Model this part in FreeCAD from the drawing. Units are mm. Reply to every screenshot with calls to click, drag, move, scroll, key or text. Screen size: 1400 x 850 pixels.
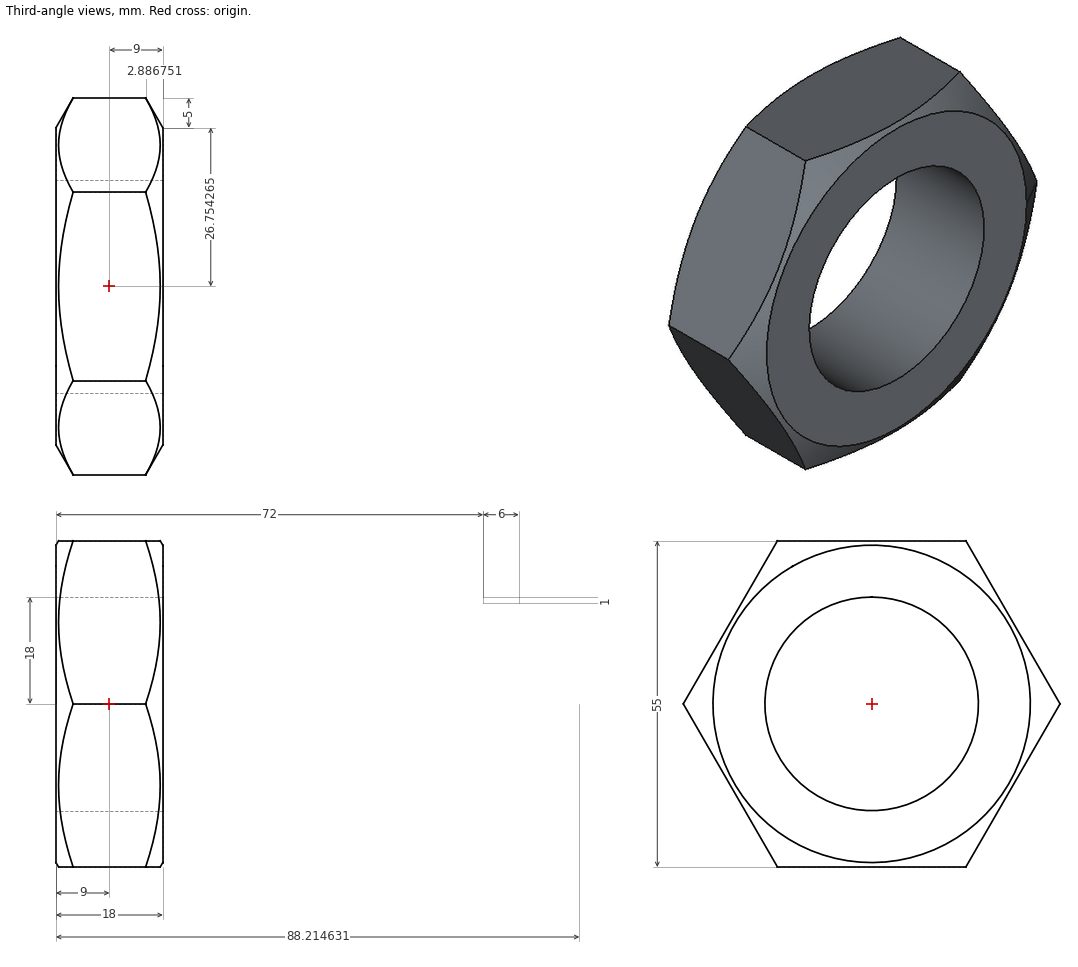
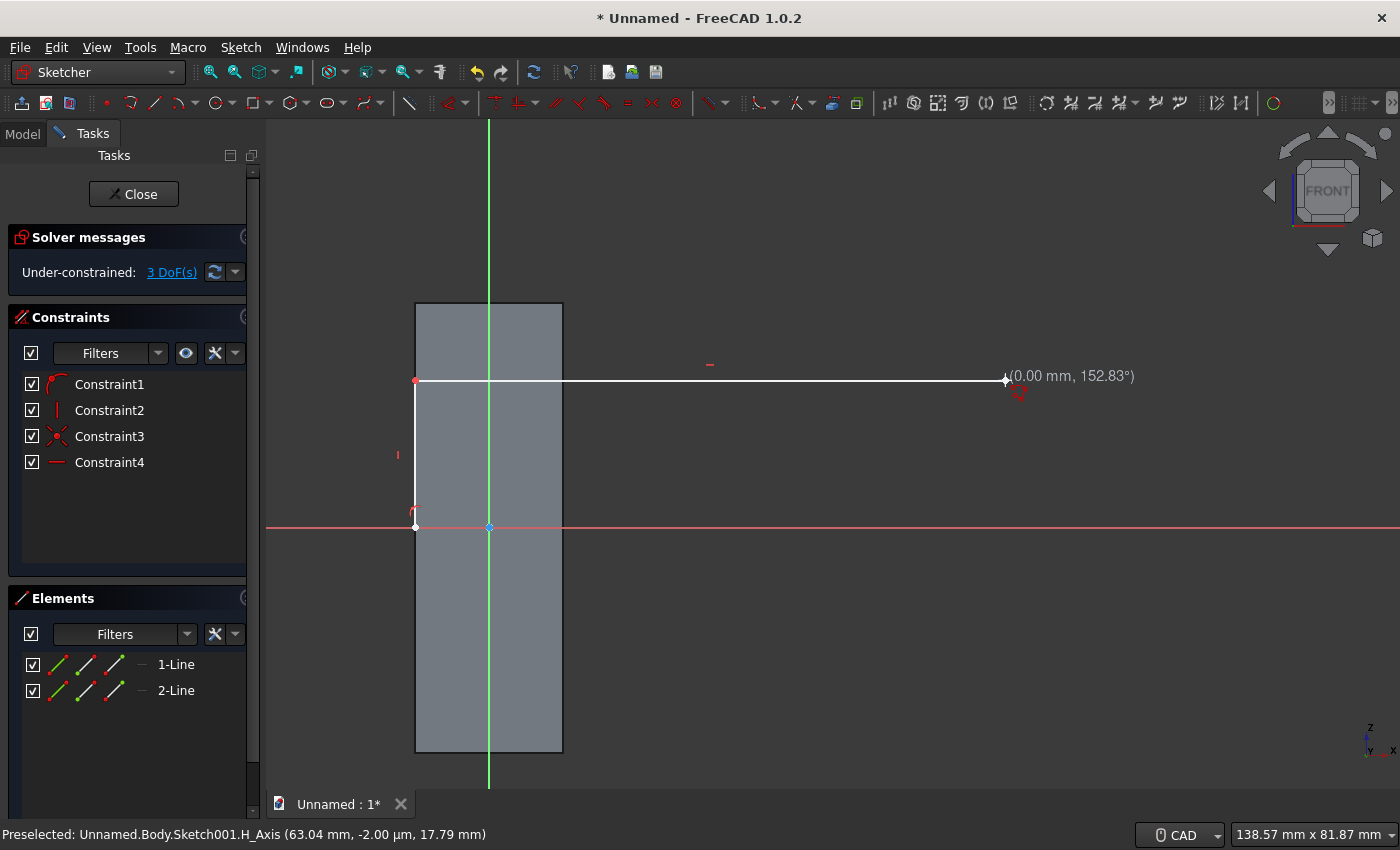
scroll(1005, 388, up, 4)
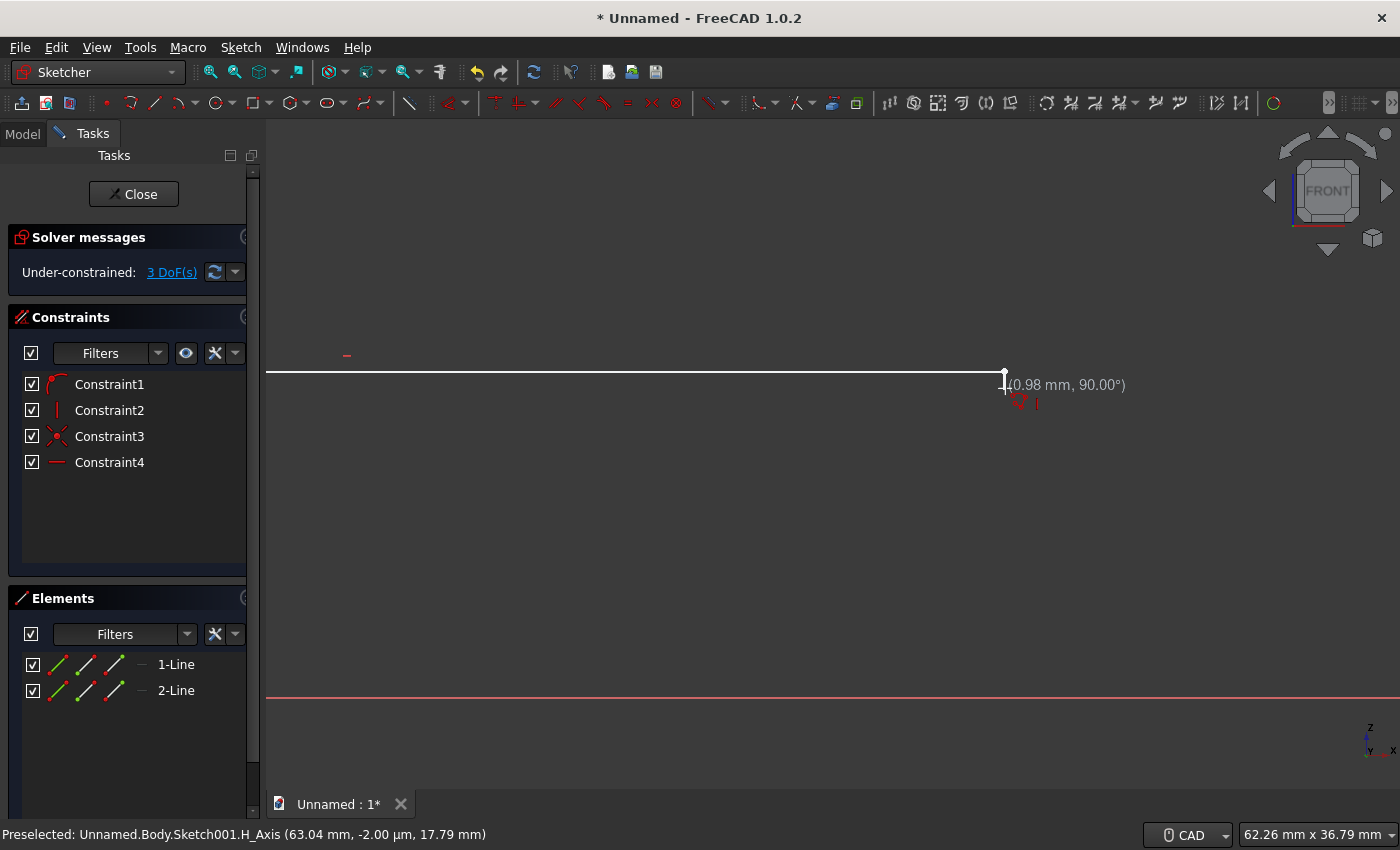
click(1004, 388)
click(1113, 388)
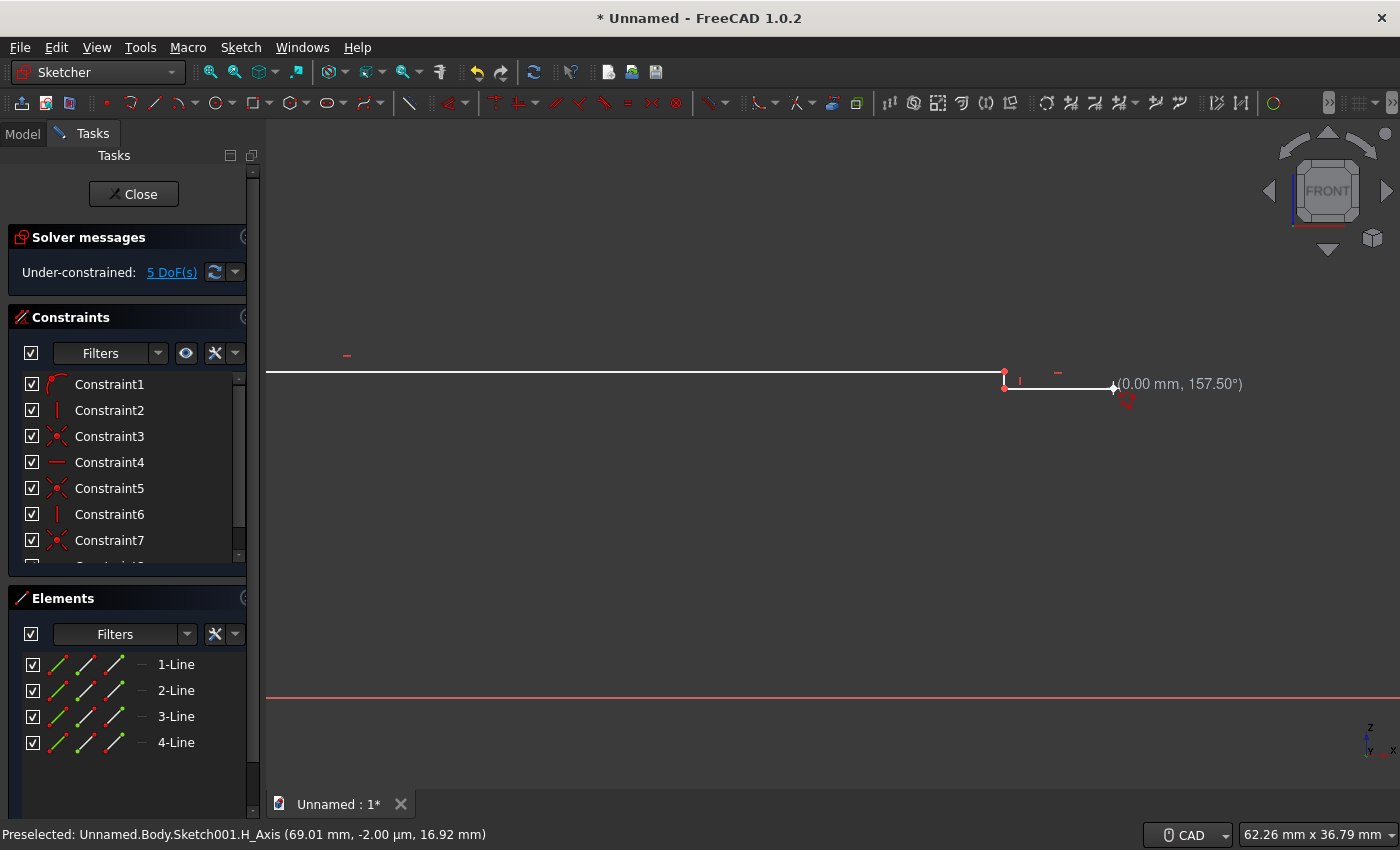
scroll(984, 389, down, 4)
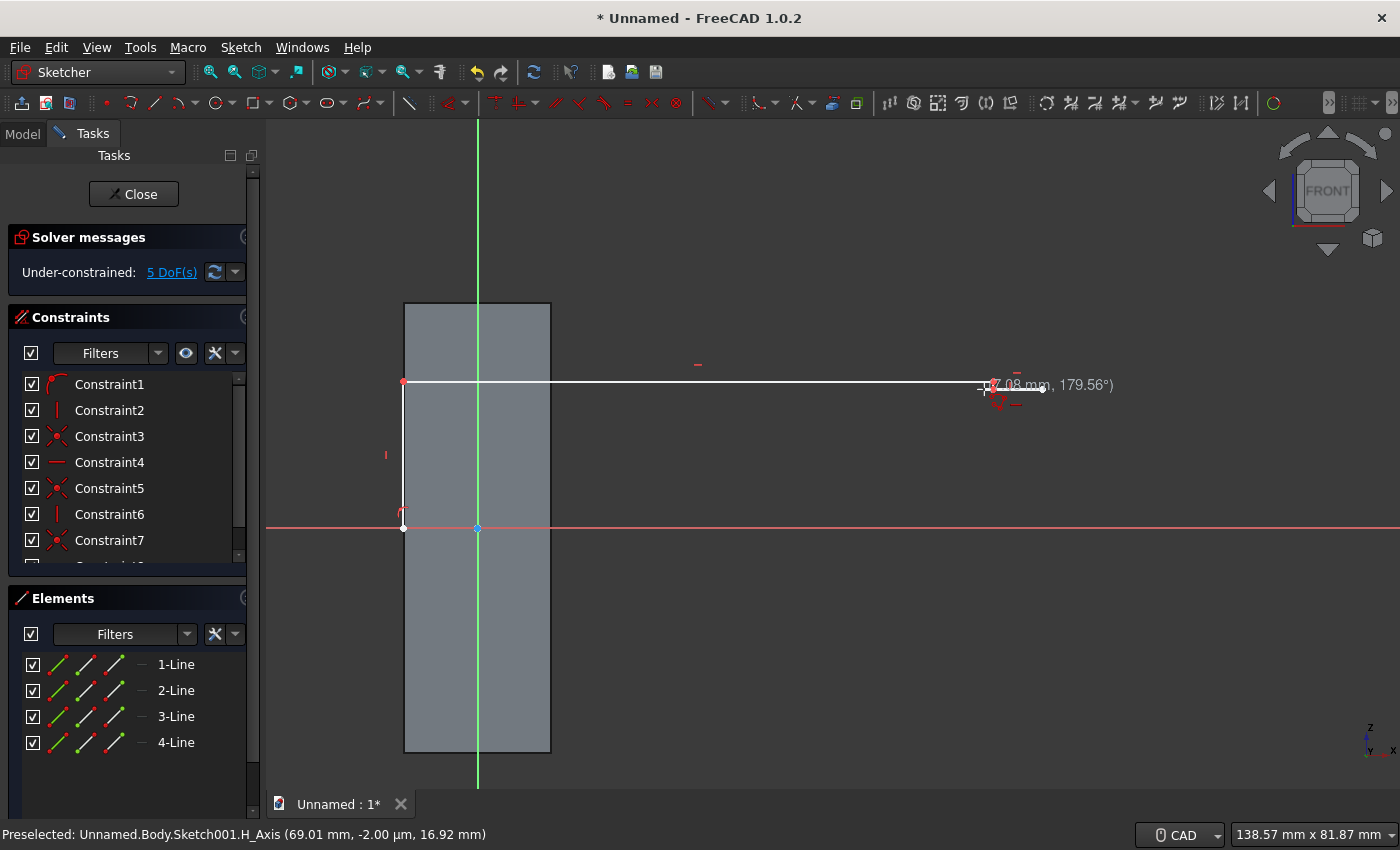
click(1126, 519)
click(403, 528)
key(Escape)
key(Escape)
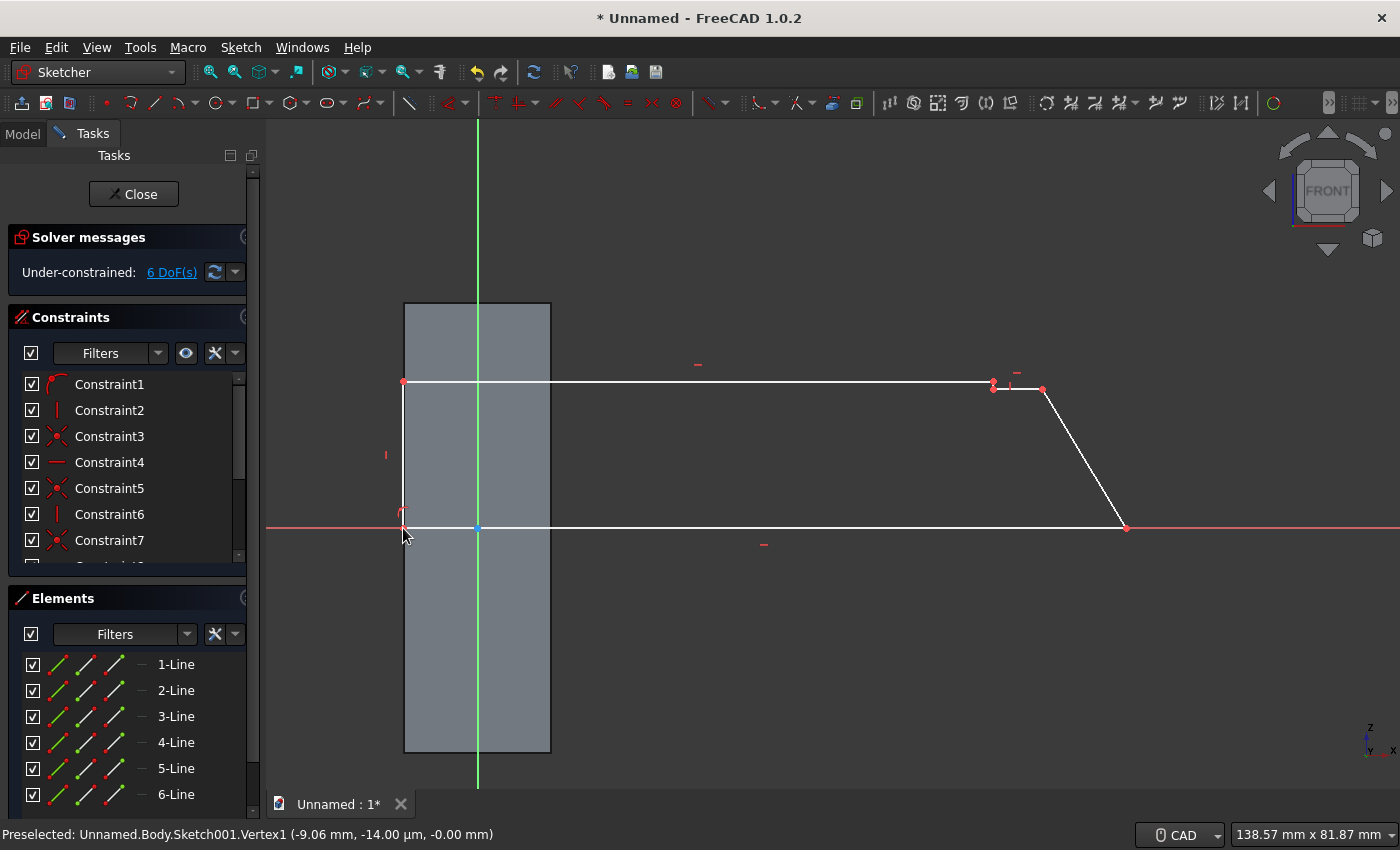
scroll(993, 385, up, 8)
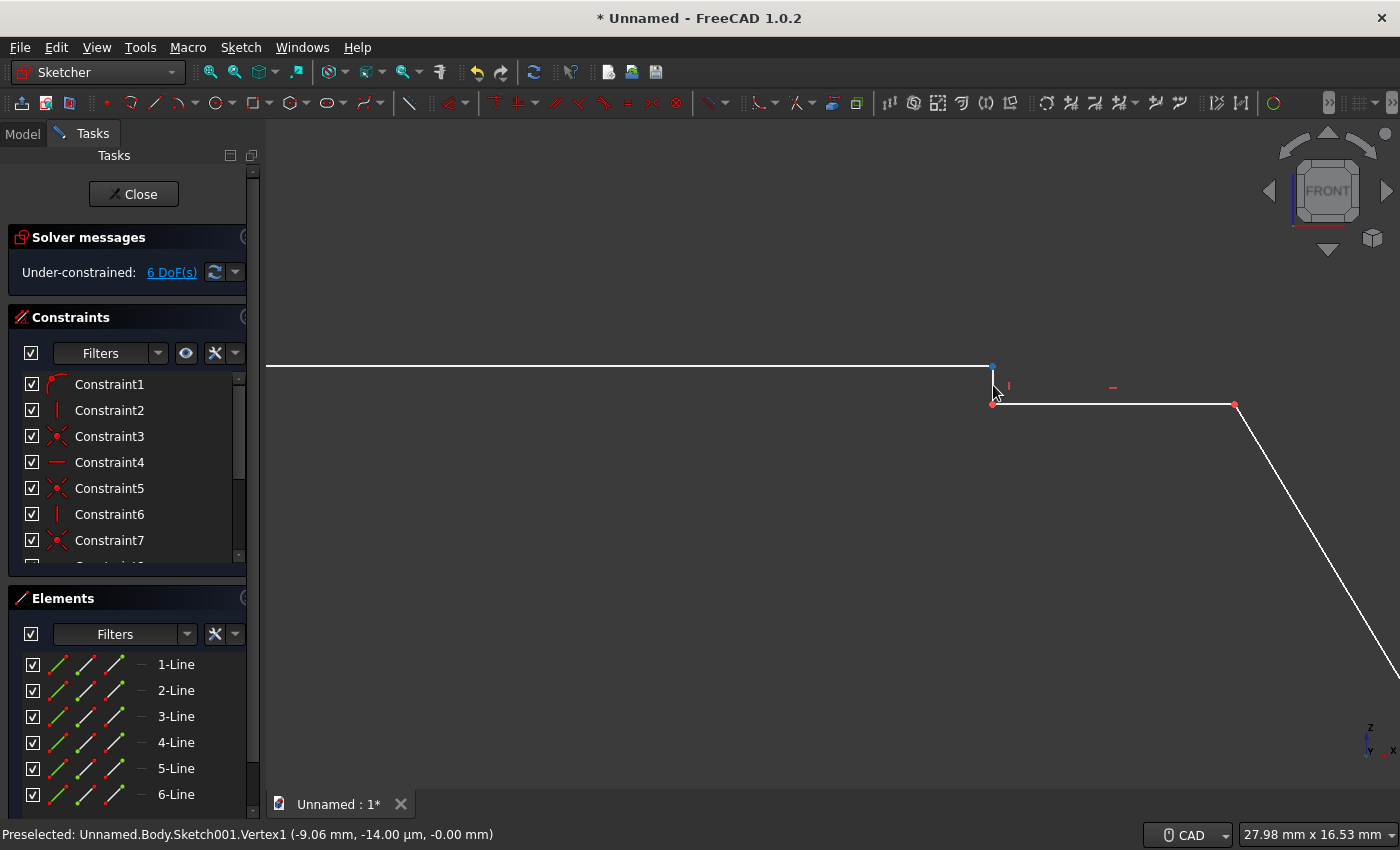
click(993, 385)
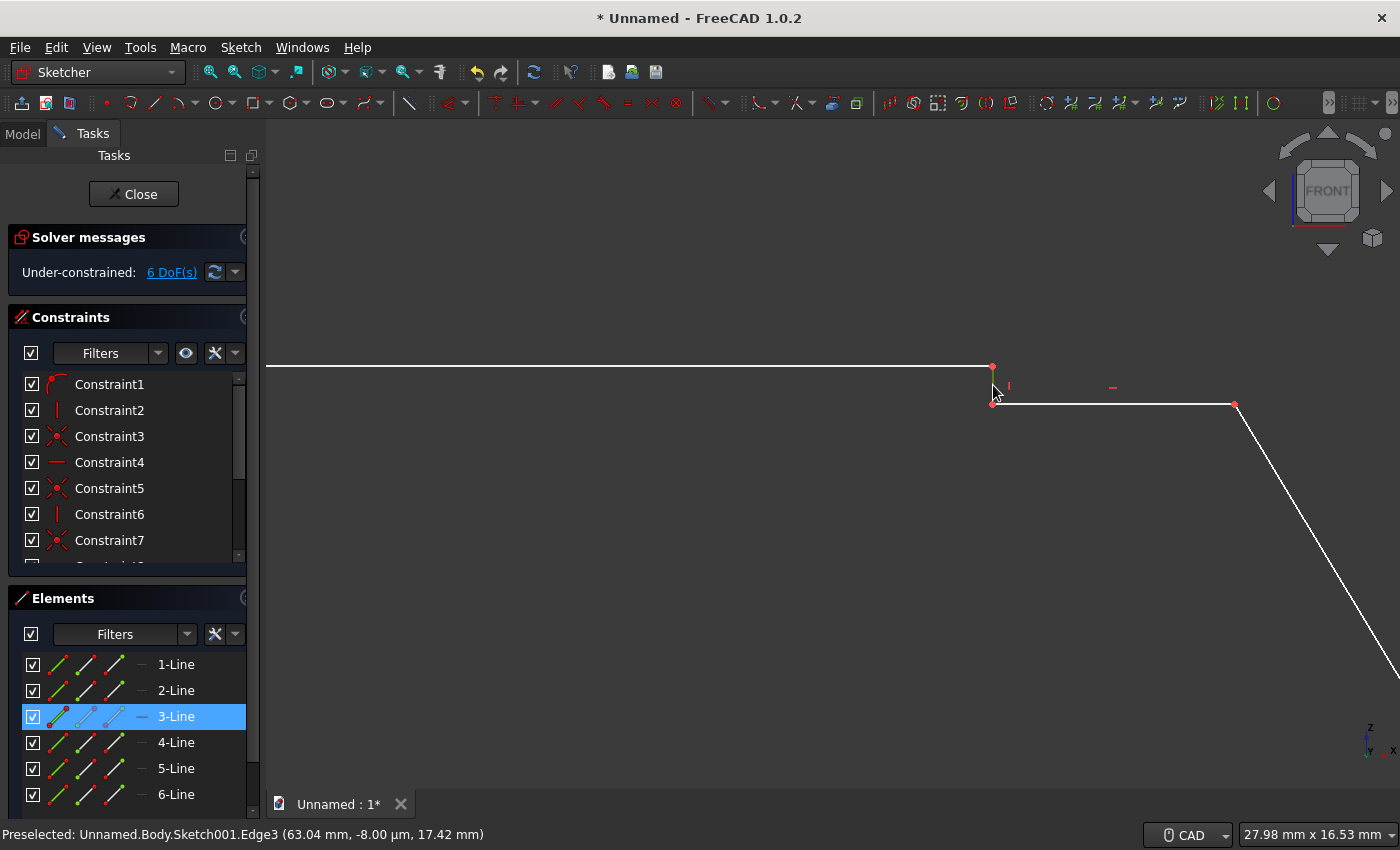
key(i)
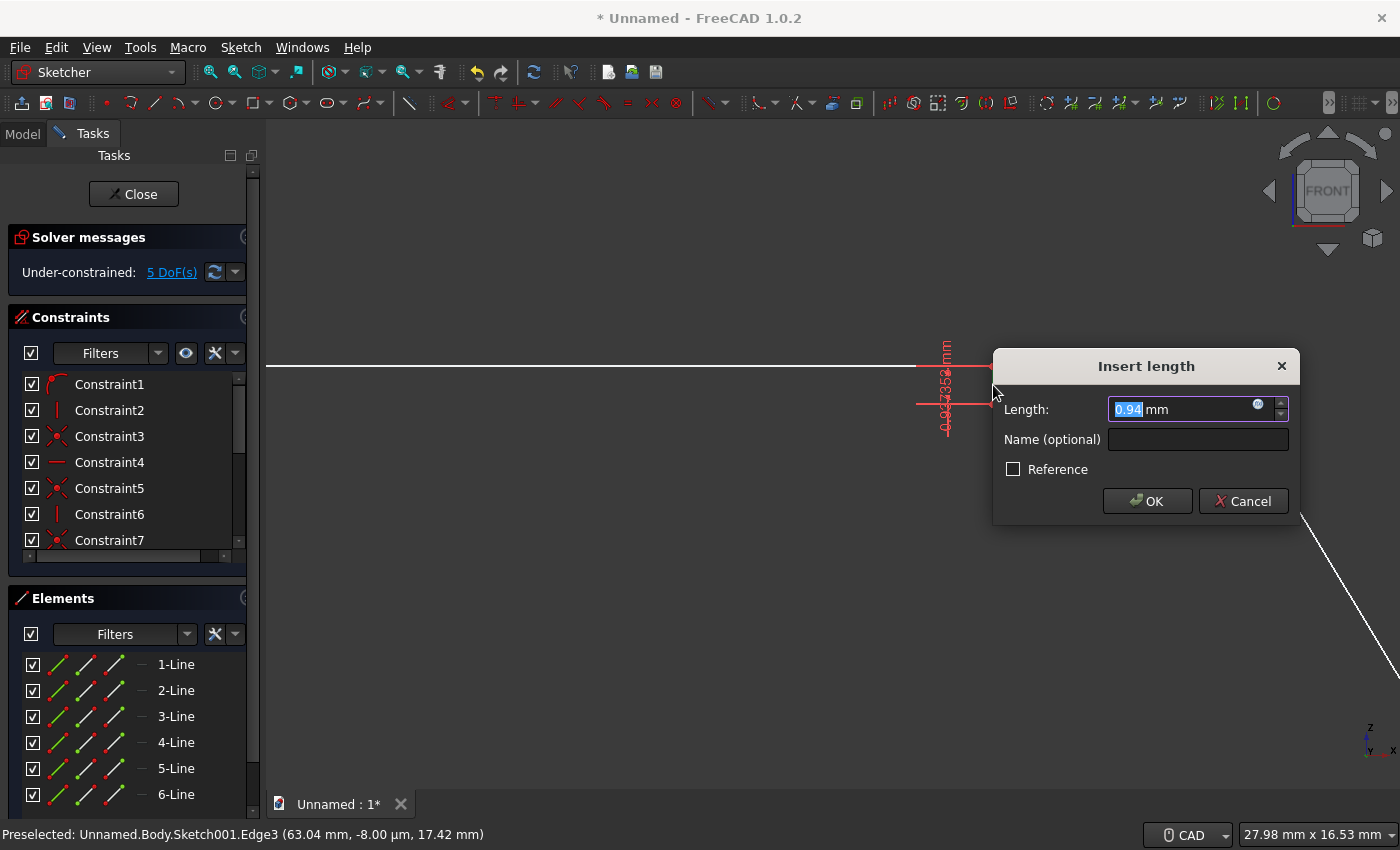
text(1)
key(Return)